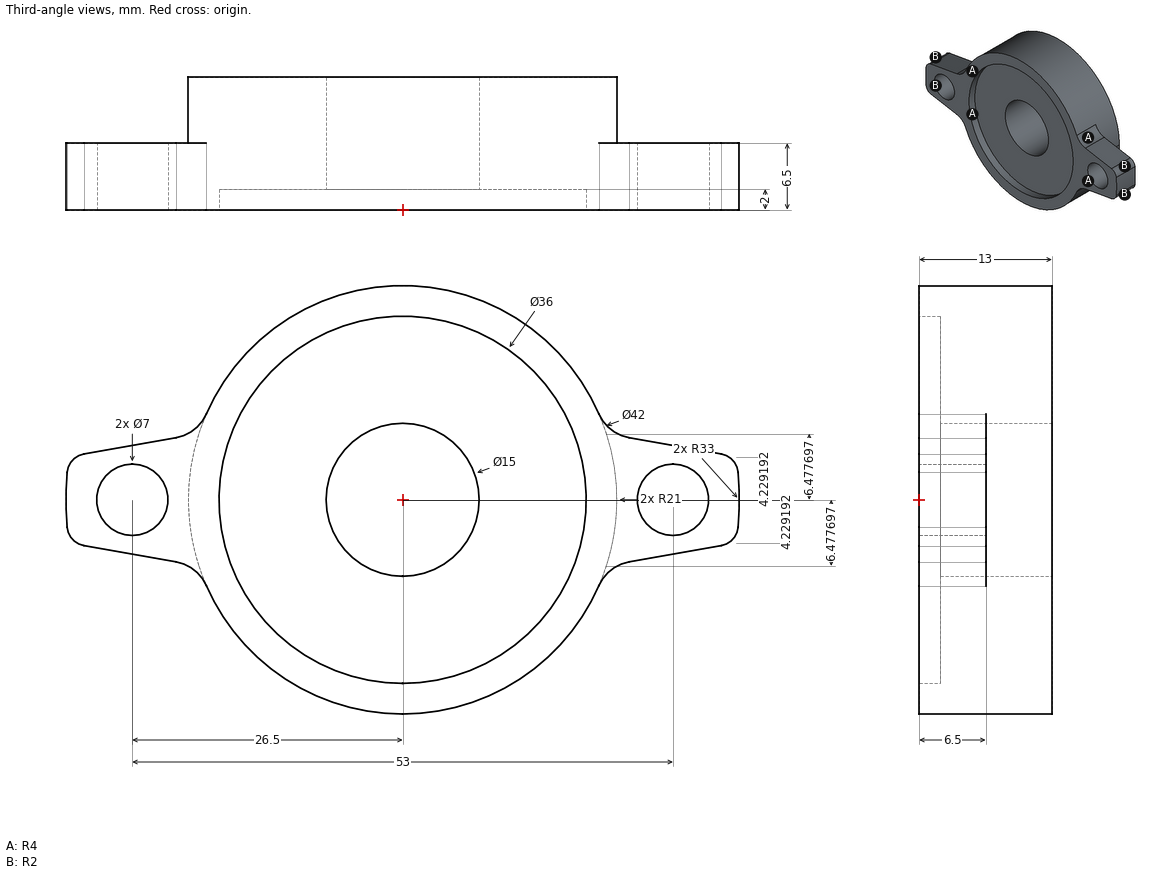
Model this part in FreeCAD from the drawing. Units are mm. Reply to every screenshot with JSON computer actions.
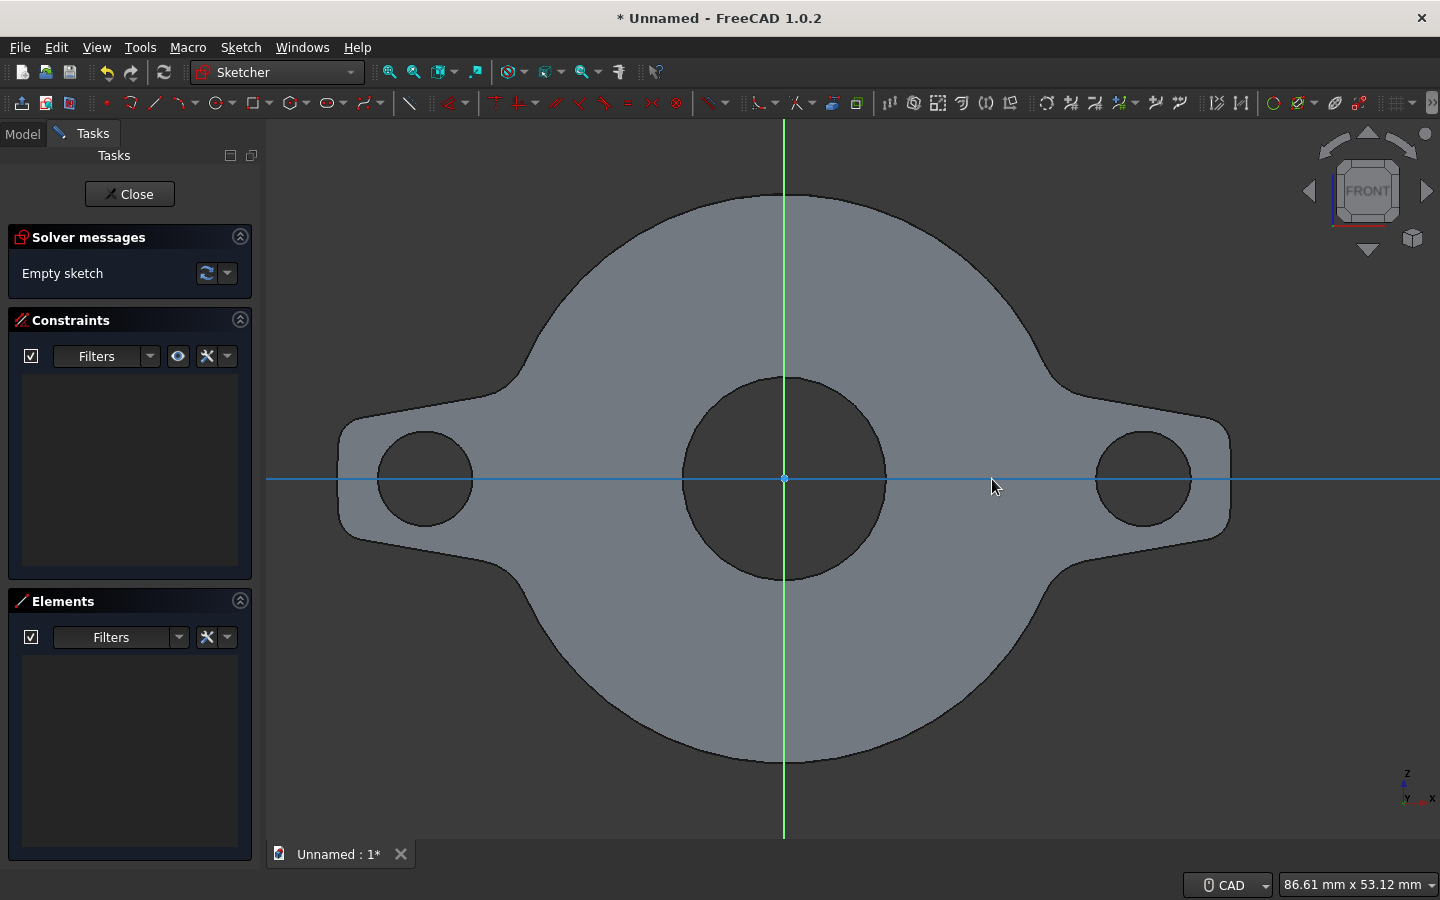
{"action": "left_click", "coordinate": [216, 104]}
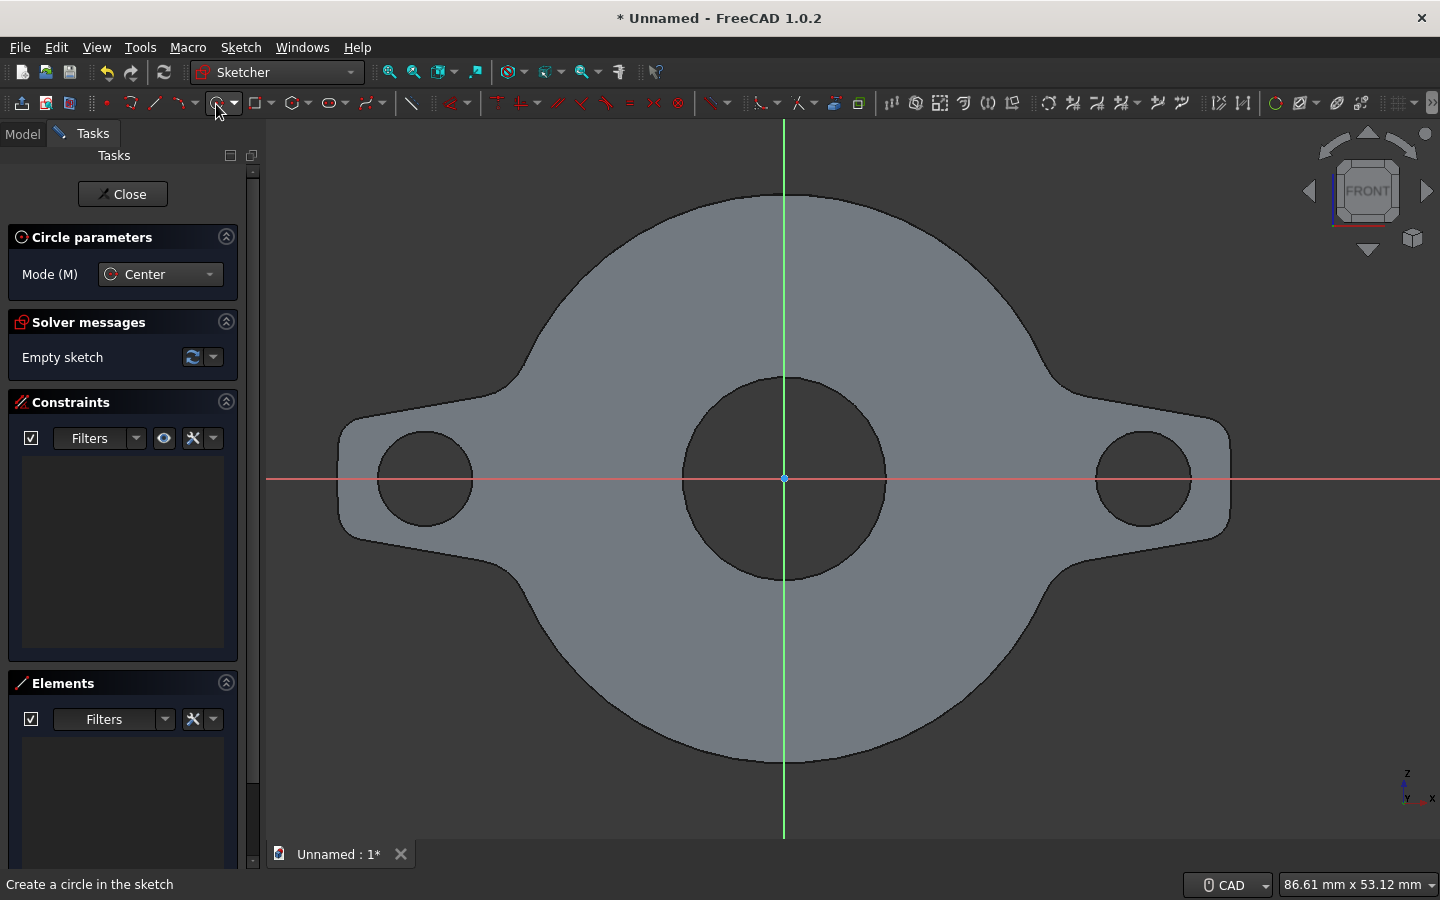
{"action": "left_click", "coordinate": [784, 479]}
{"action": "mouse_move", "coordinate": [957, 306]}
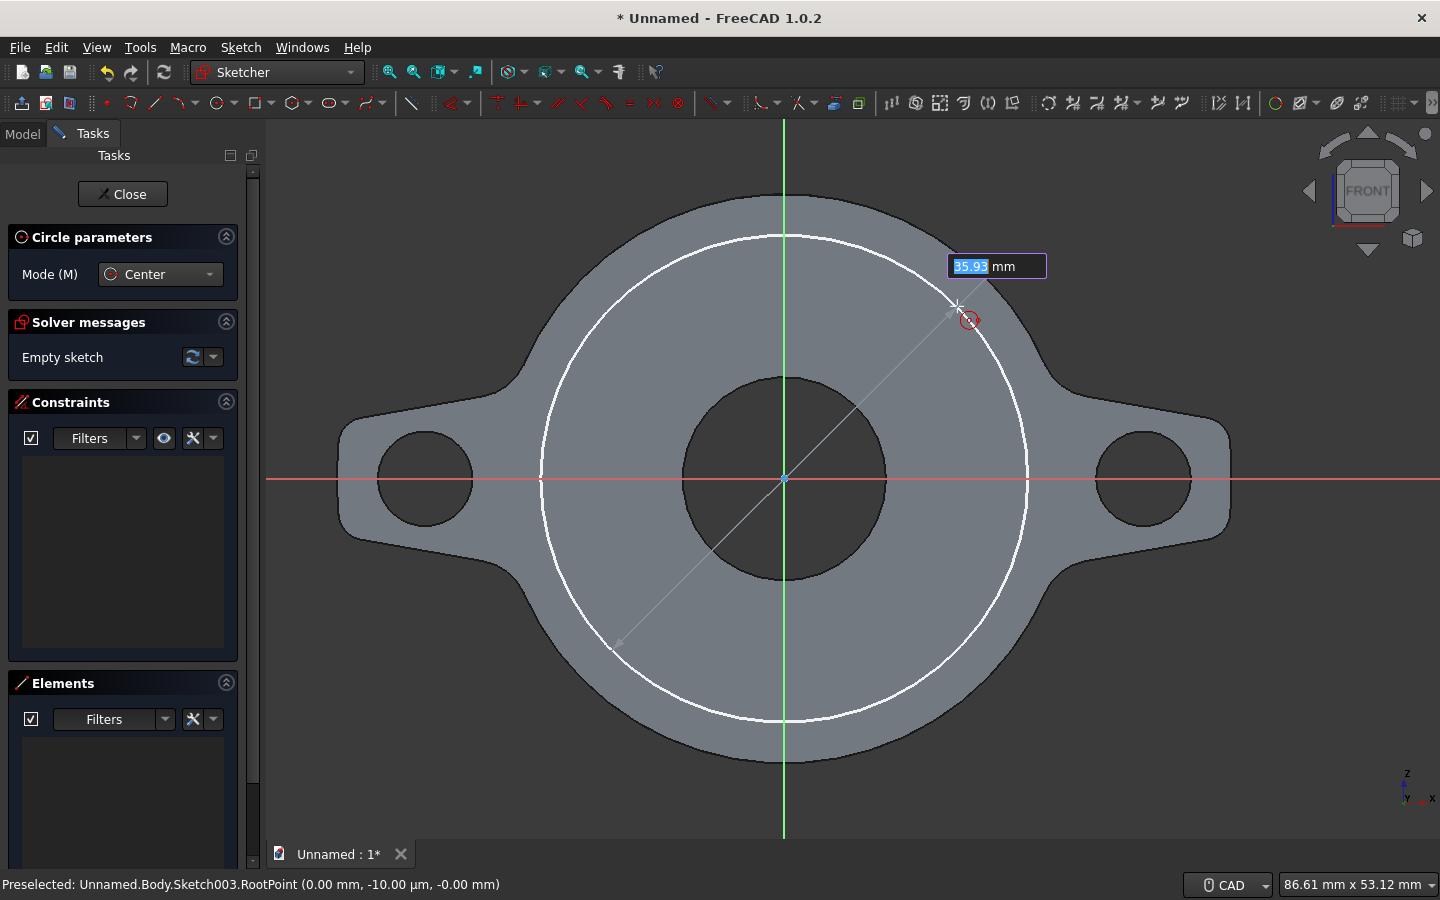
{"action": "type", "text": "36"}
{"action": "key", "text": "Return"}
{"action": "key", "text": "Escape"}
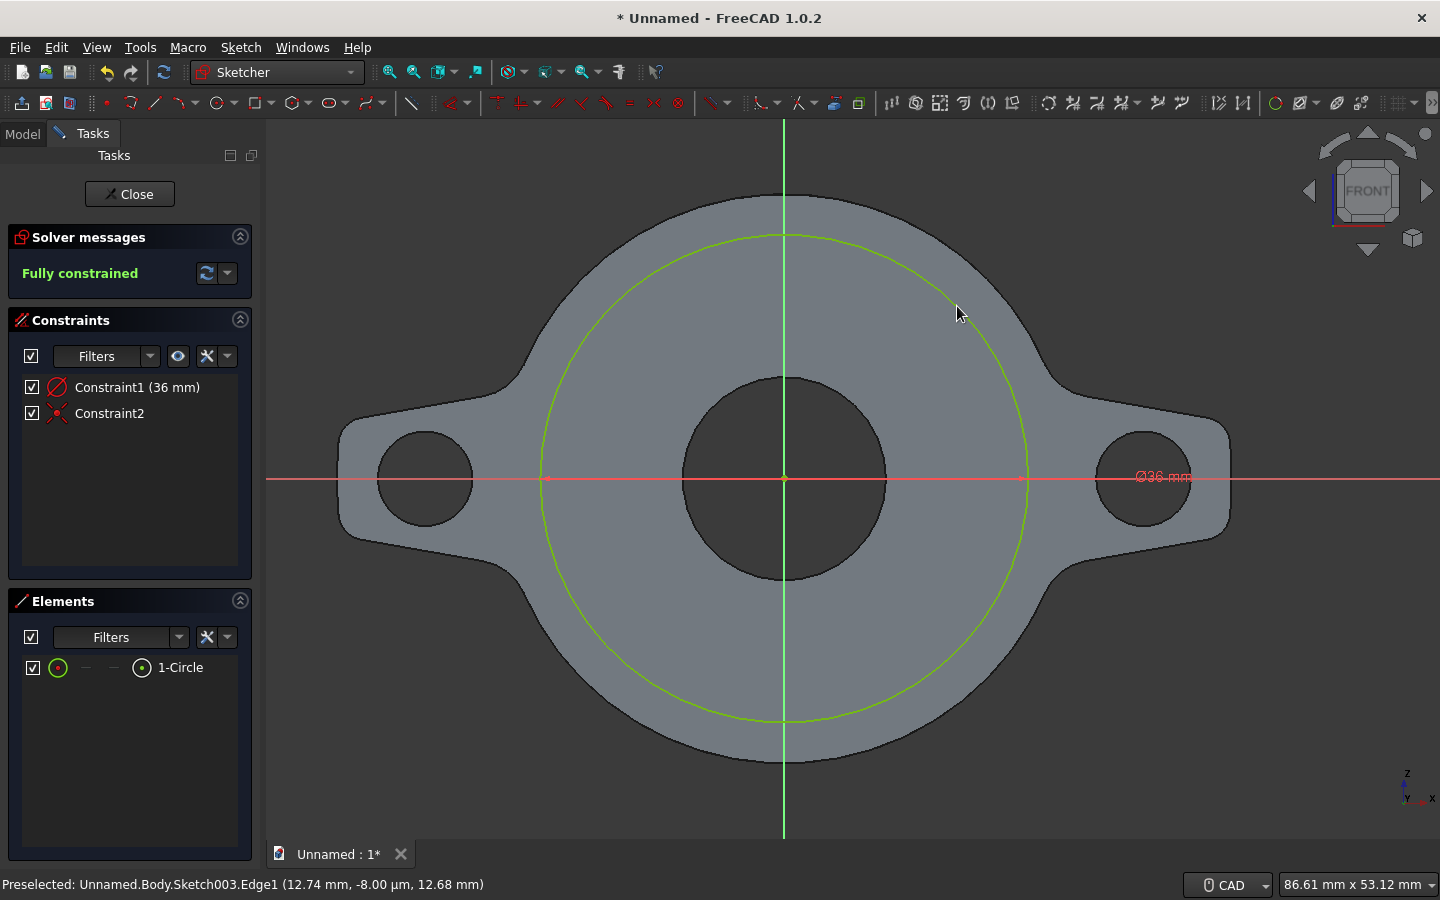
{"action": "left_click", "coordinate": [130, 194]}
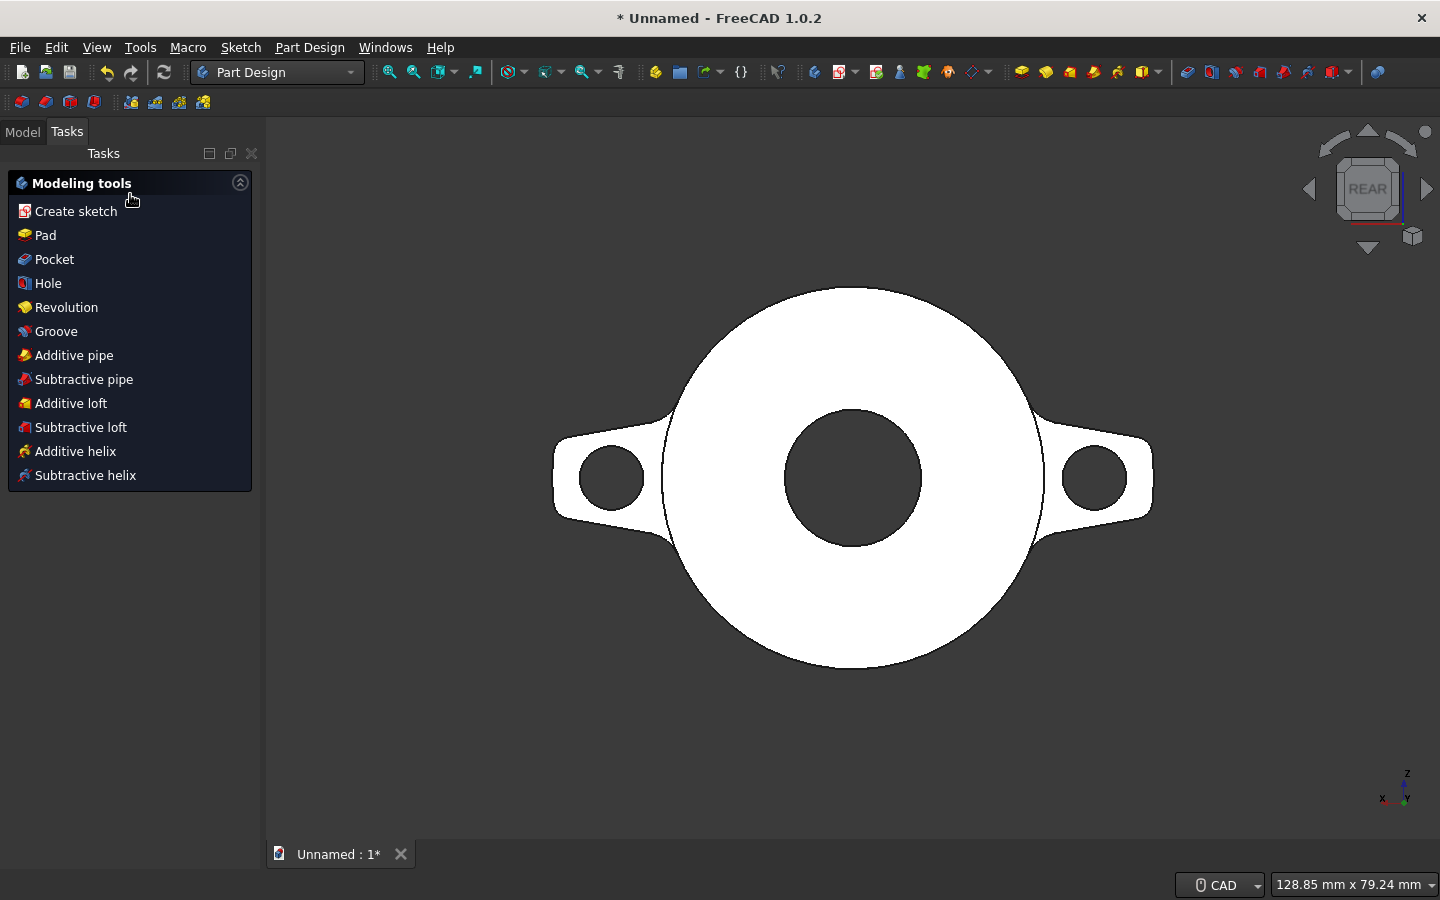
{"action": "left_click", "coordinate": [1188, 72]}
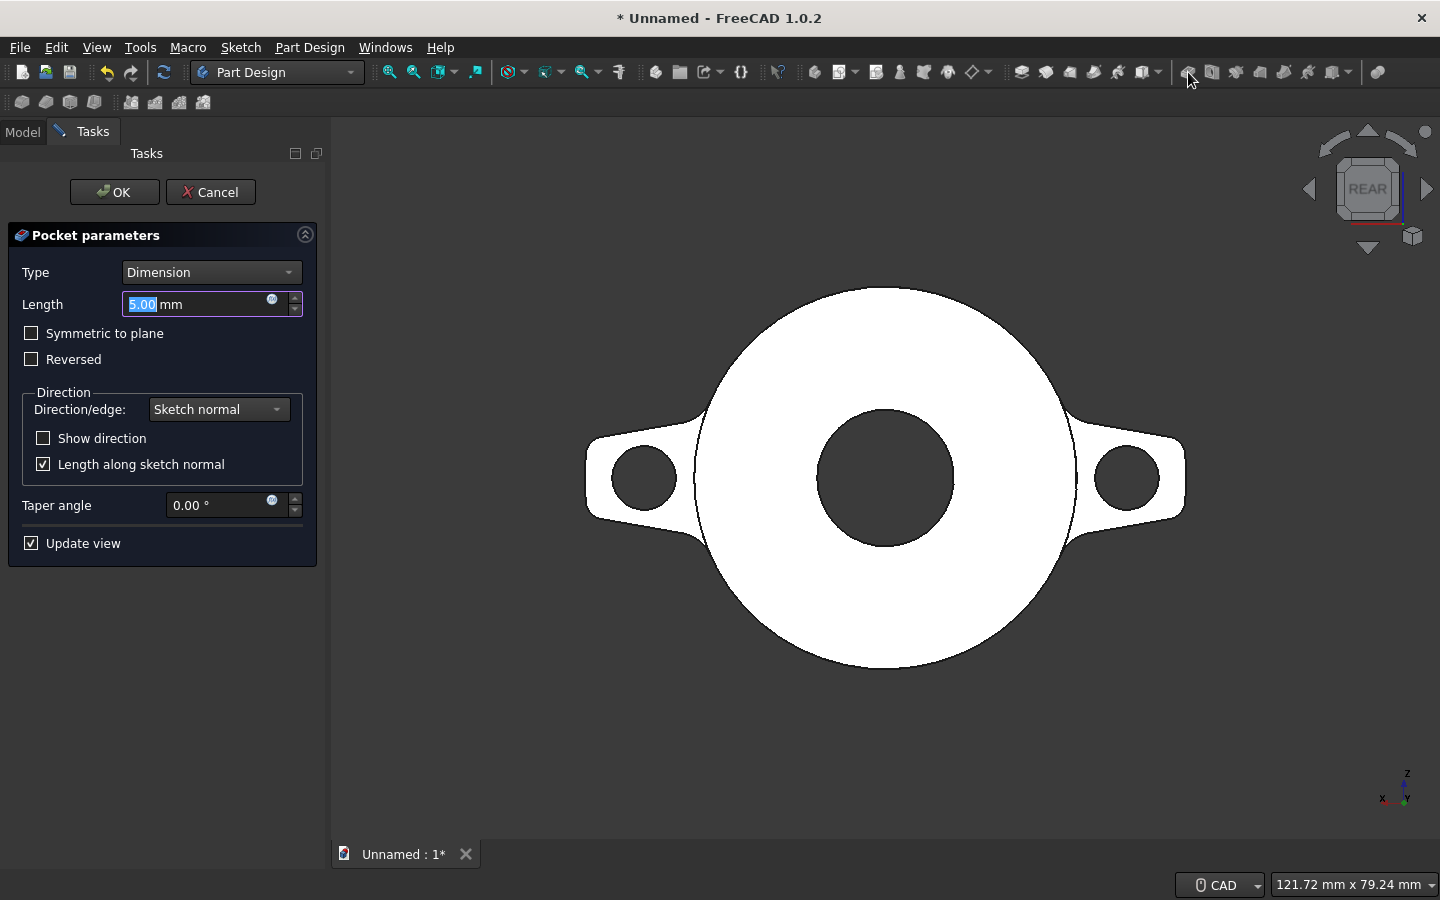
{"action": "type", "text": "2"}
{"action": "key", "text": "Tab"}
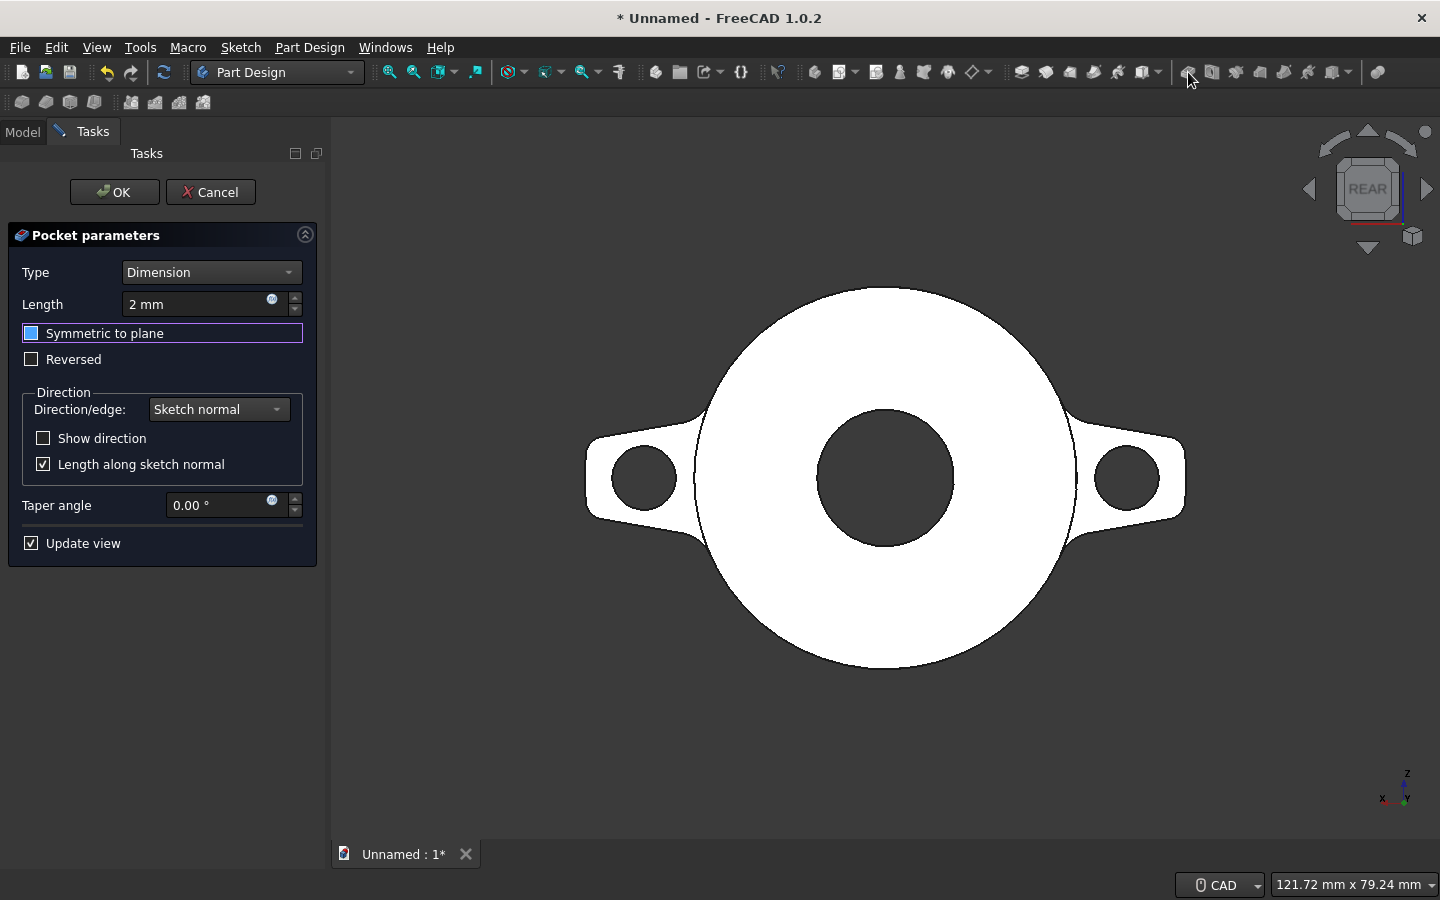
{"action": "left_click", "coordinate": [115, 192]}